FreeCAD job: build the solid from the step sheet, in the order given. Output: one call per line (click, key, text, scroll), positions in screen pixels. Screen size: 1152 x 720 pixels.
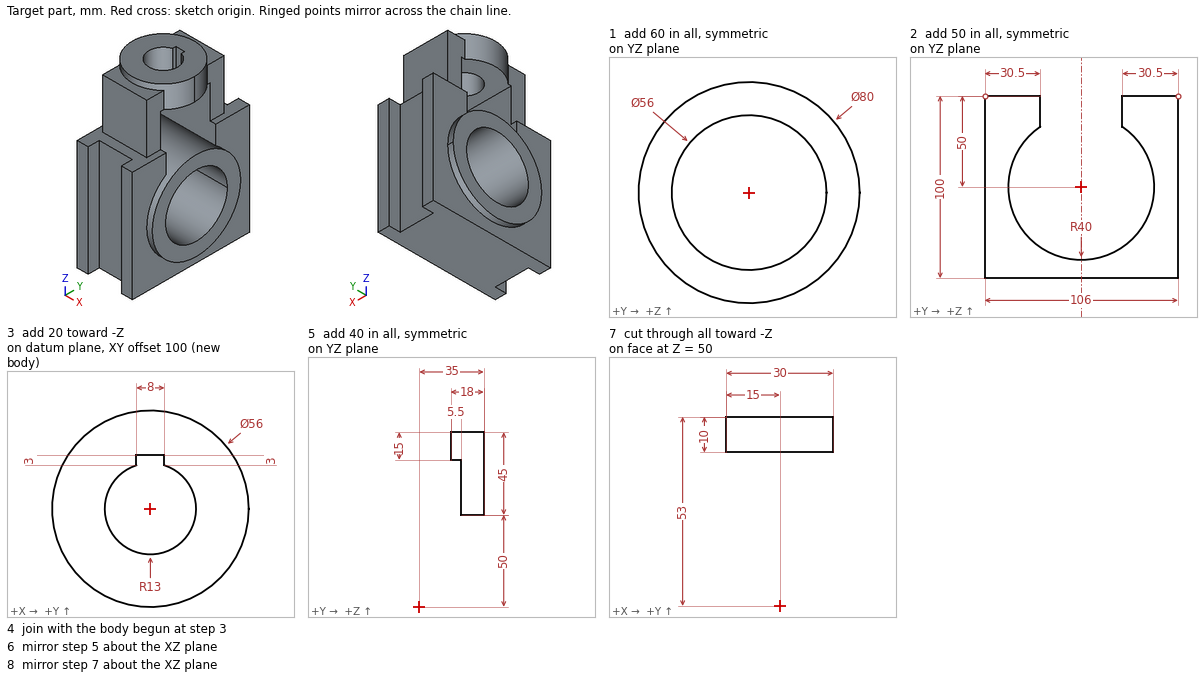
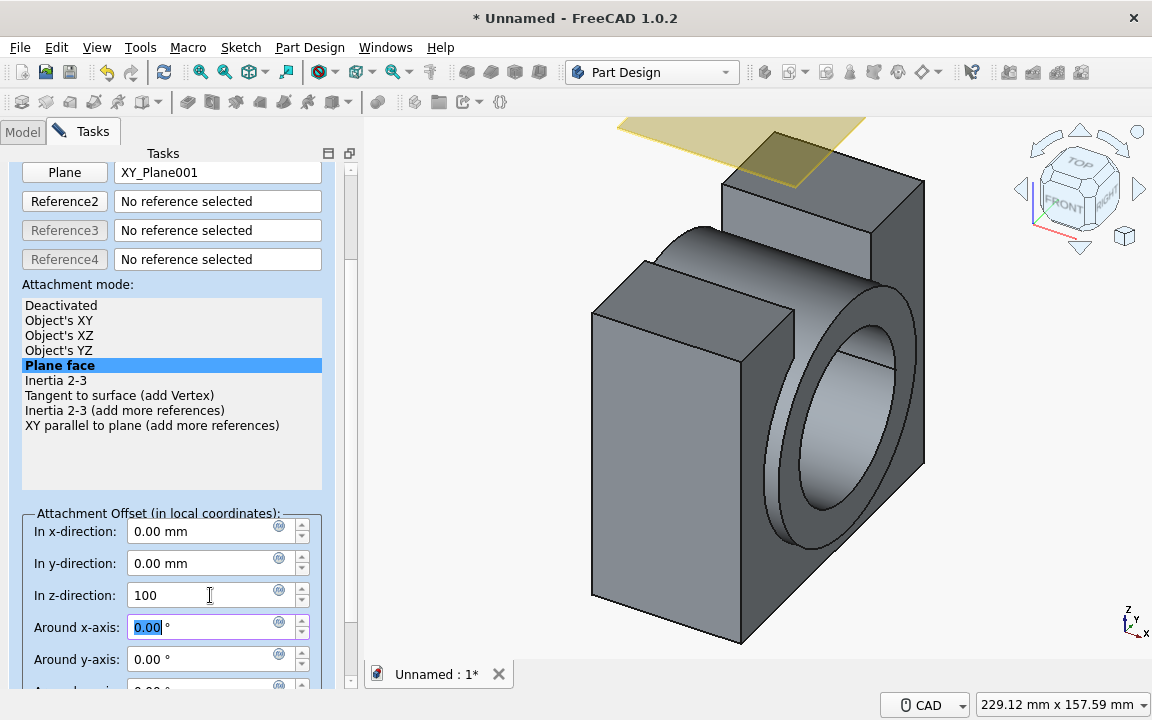
scroll(351, 426, up, 3)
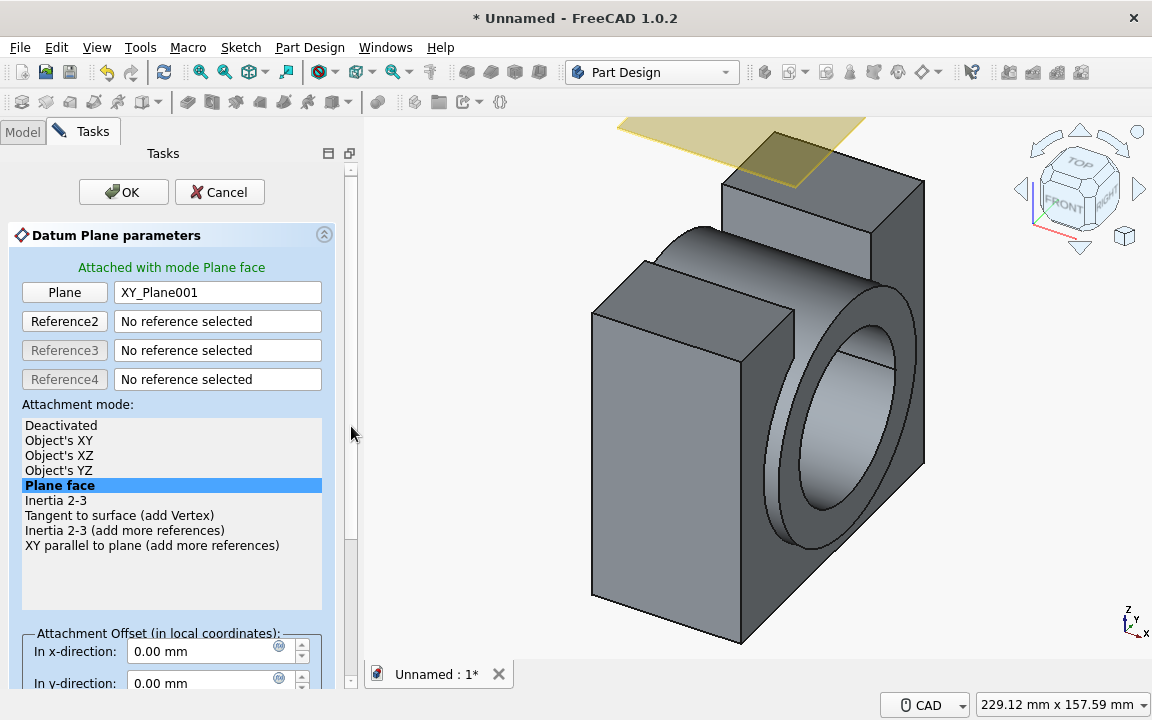
click(124, 192)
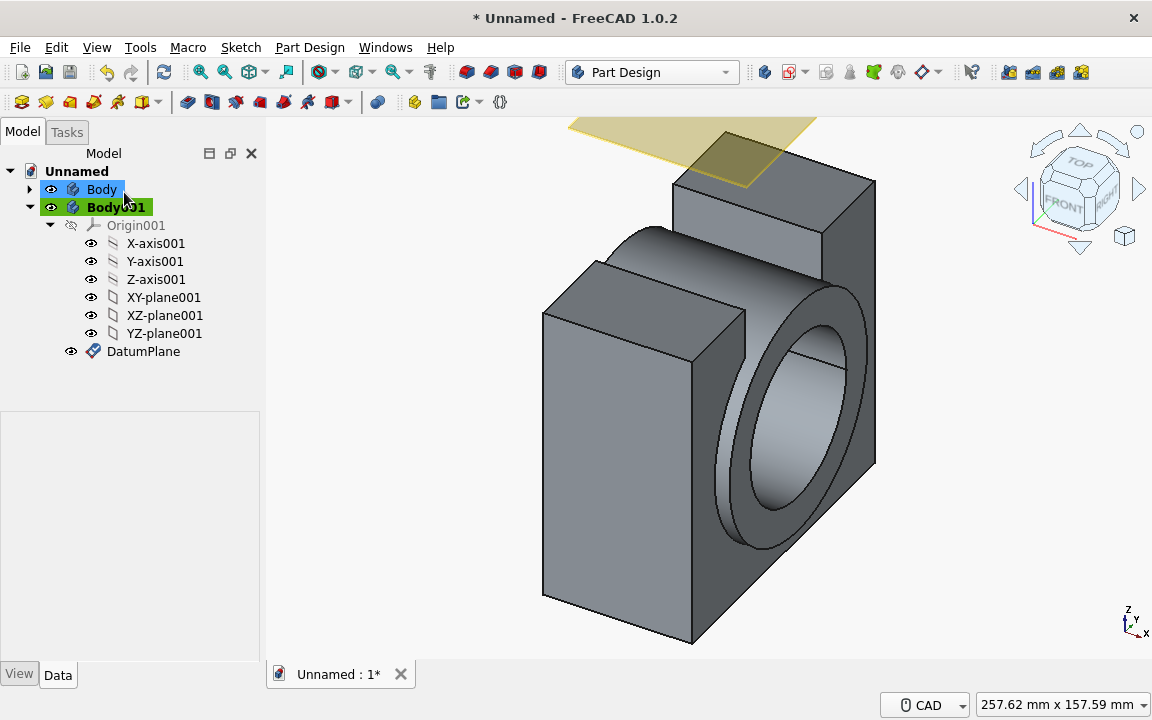
click(116, 351)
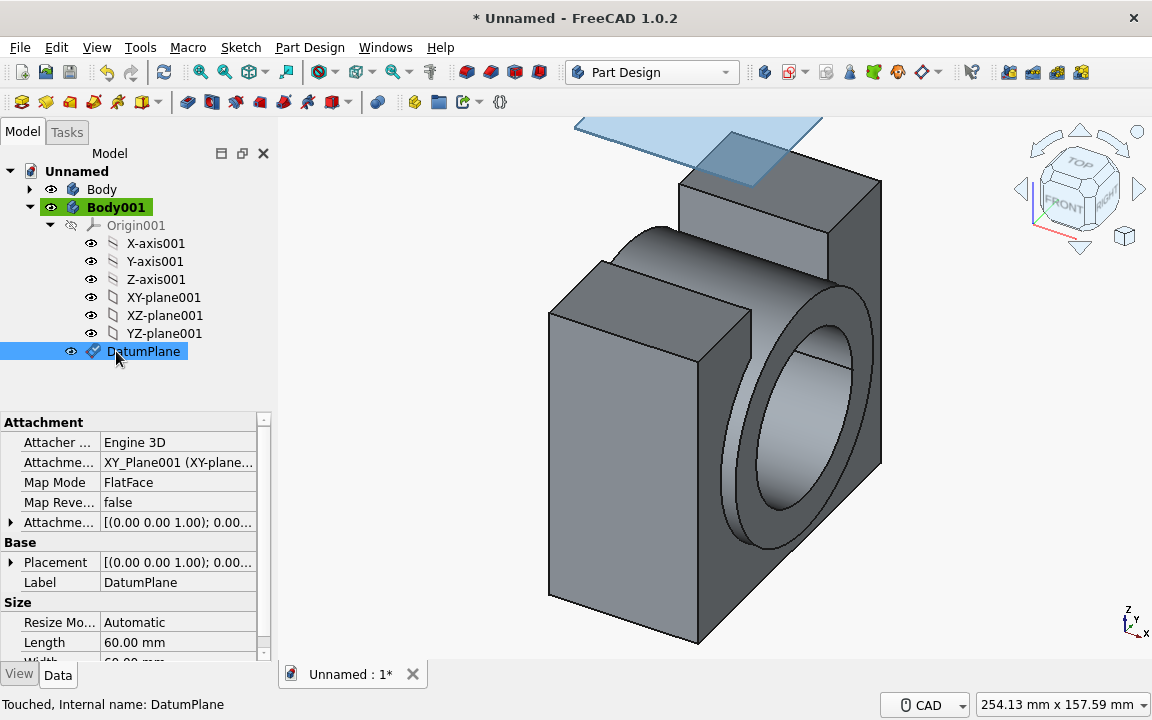
click(790, 72)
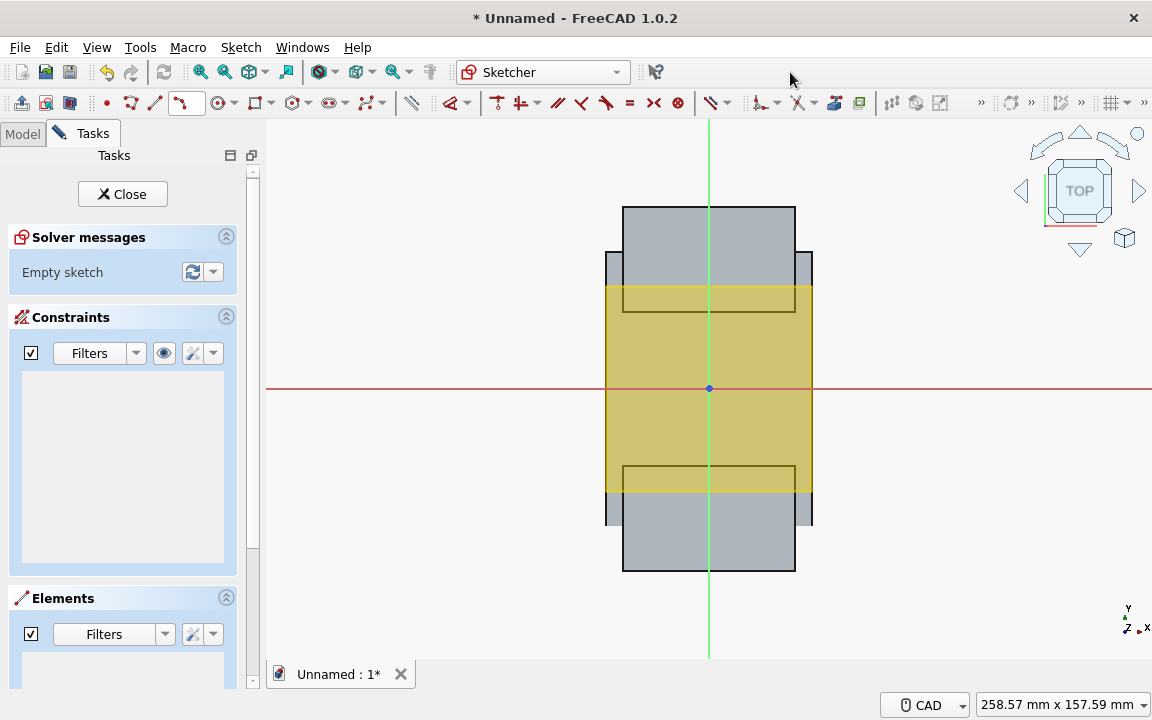
scroll(792, 389, up, 3)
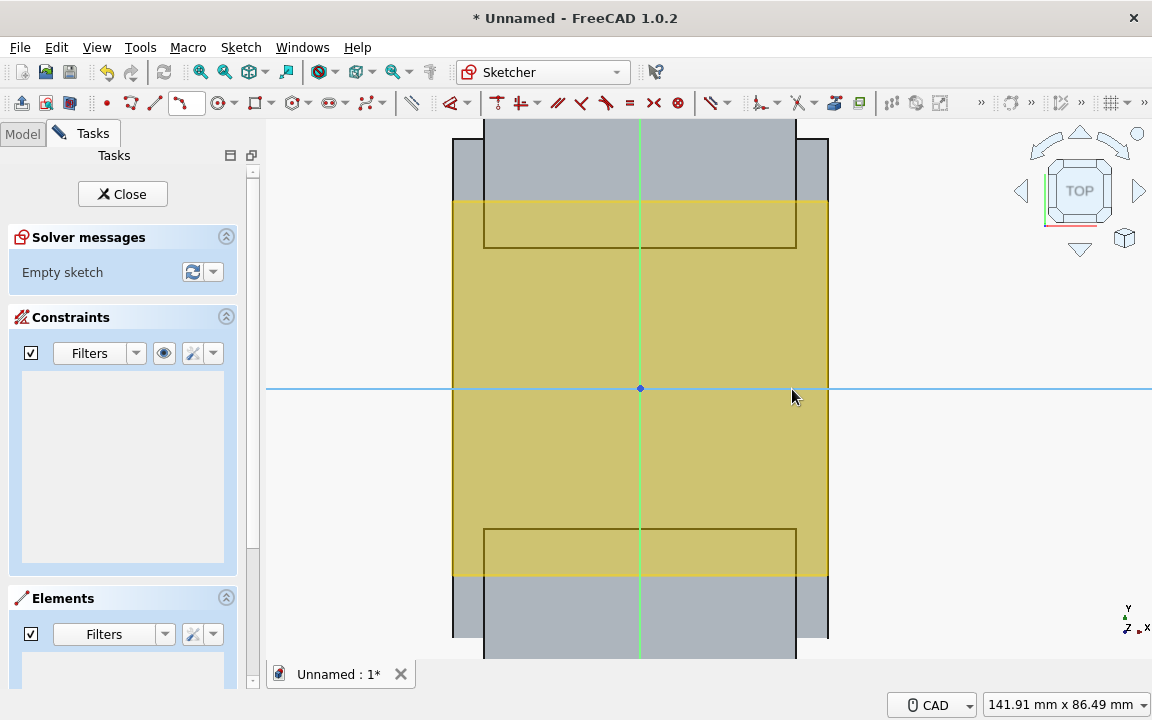
click(132, 104)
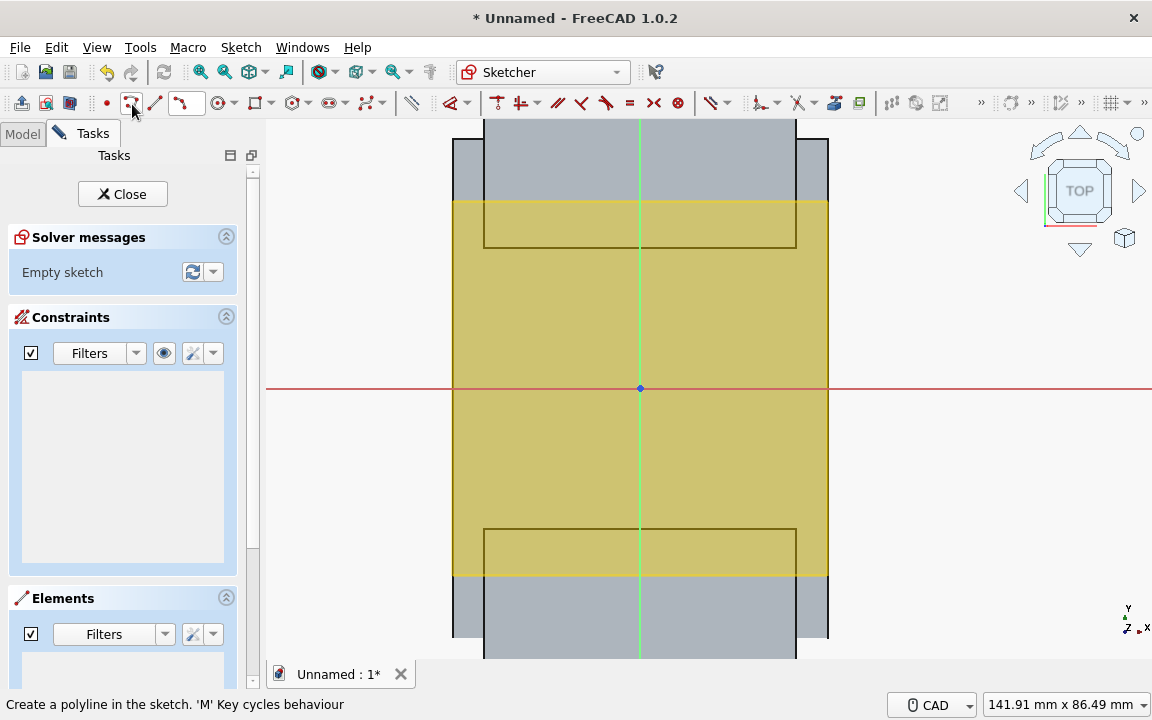
click(615, 311)
click(615, 293)
click(665, 293)
click(665, 311)
right_click(665, 311)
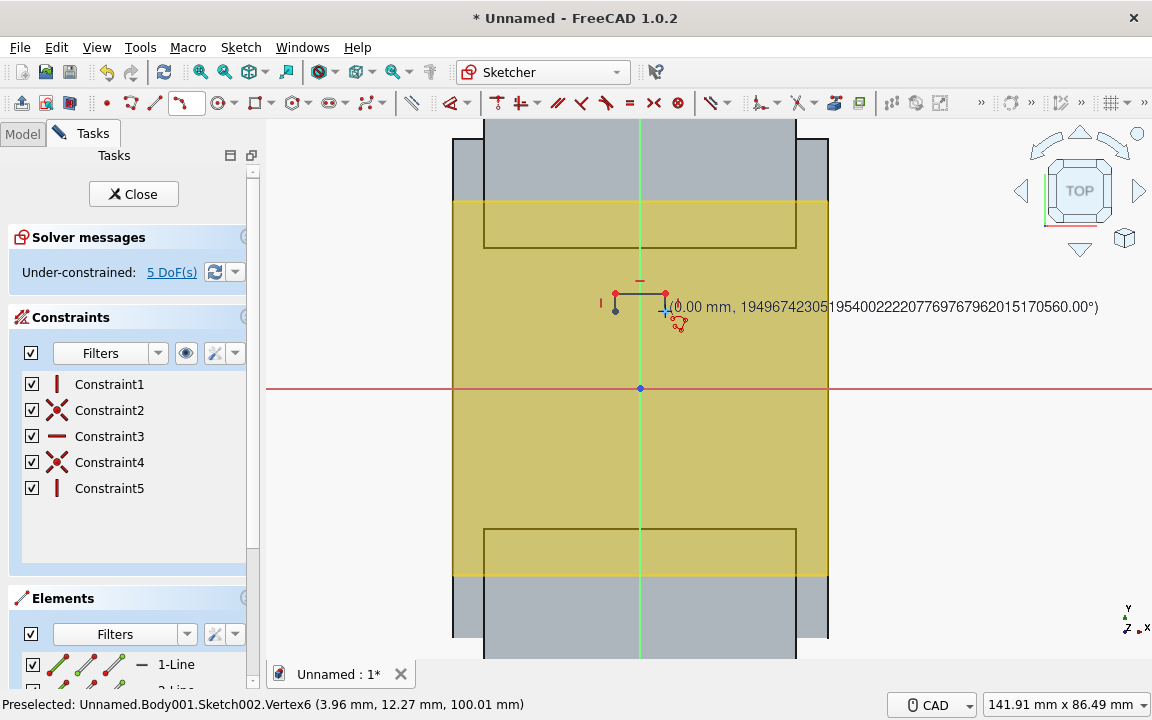
click(180, 104)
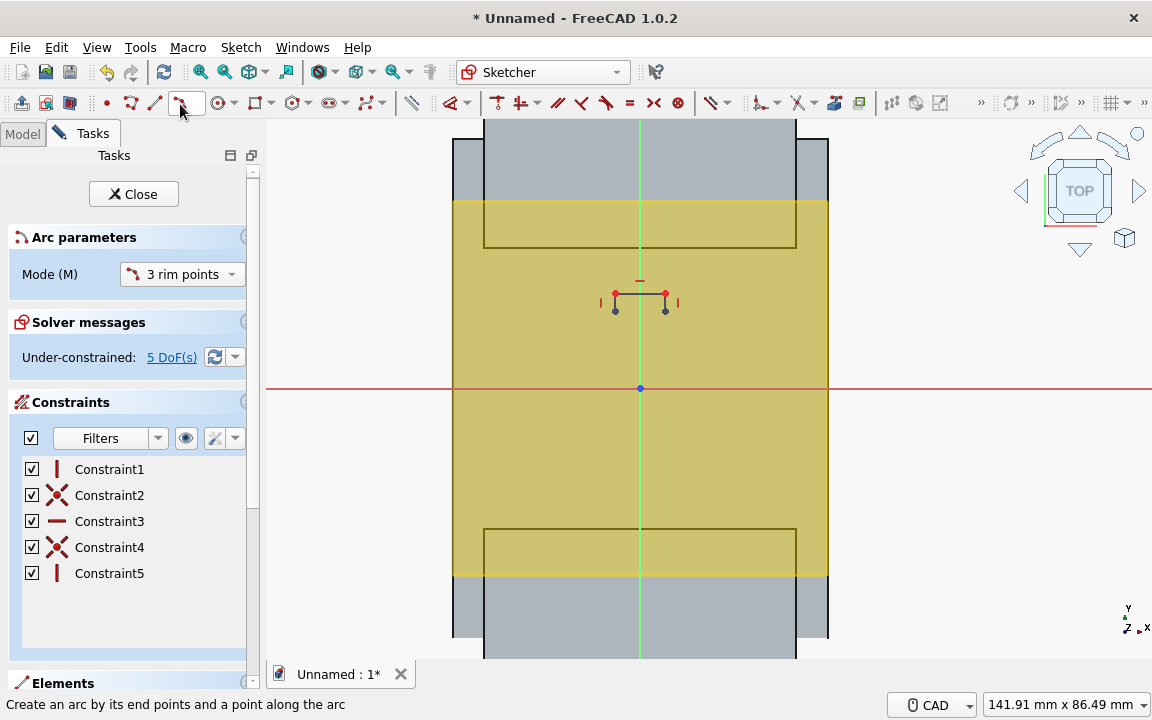
scroll(665, 311, up, 3)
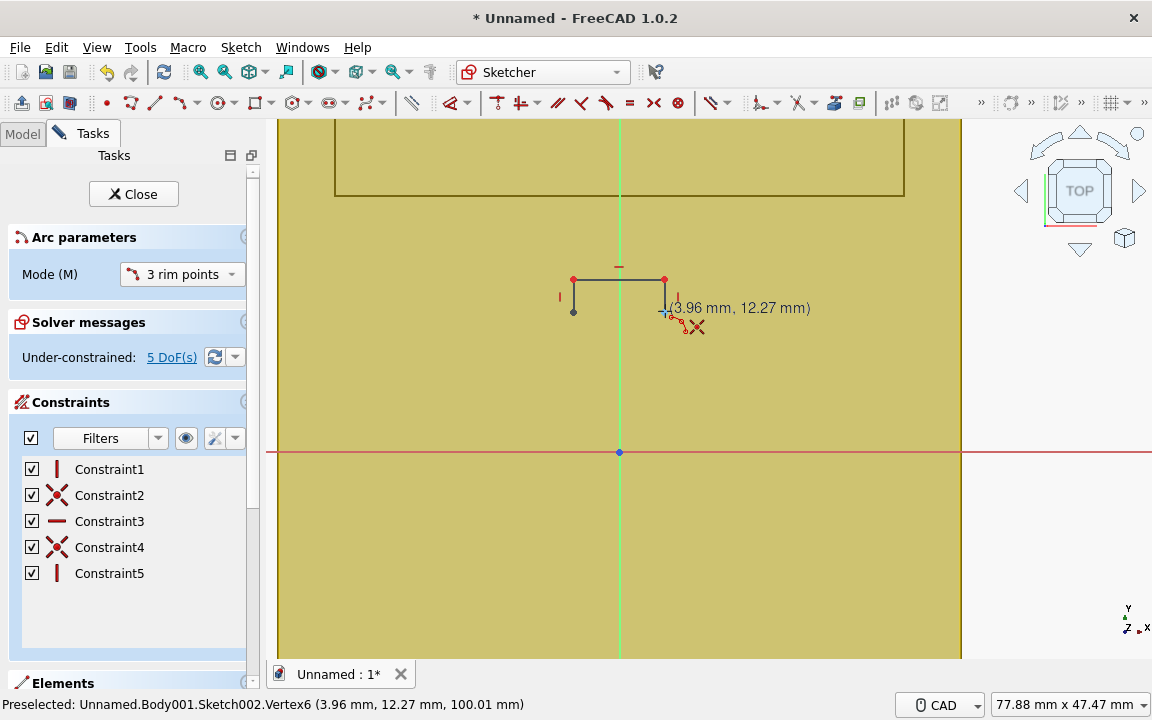
click(665, 313)
click(574, 313)
click(540, 577)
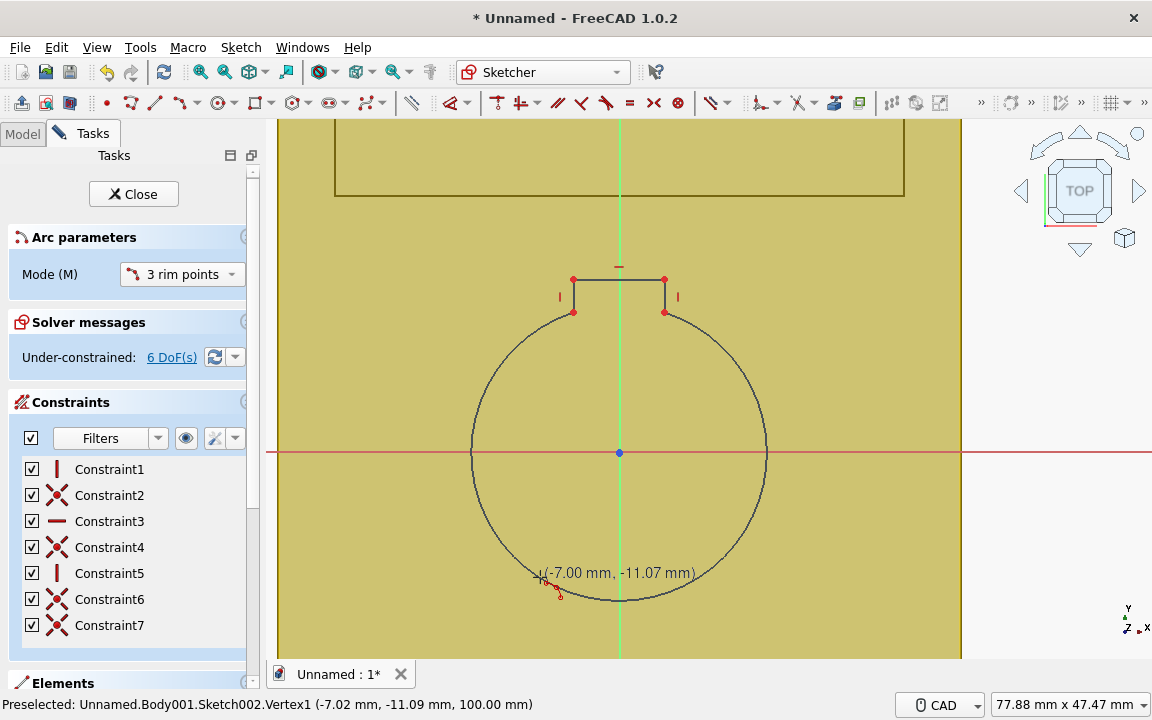
click(218, 104)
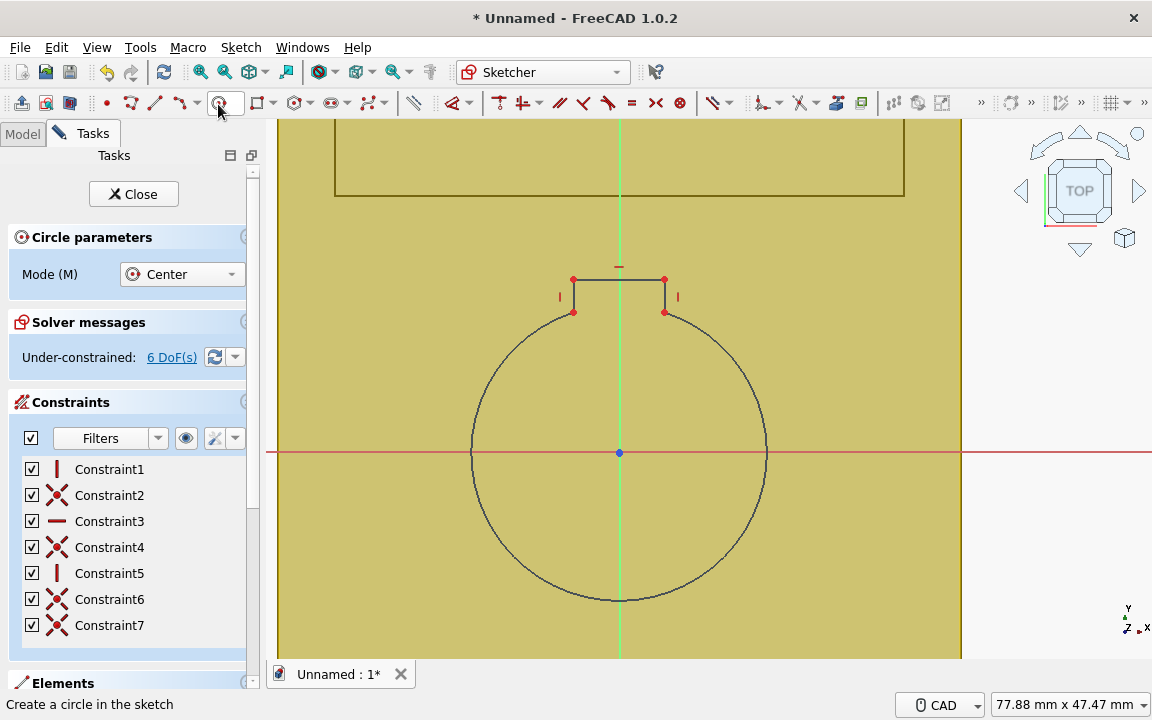
click(620, 452)
click(845, 227)
key(Escape)